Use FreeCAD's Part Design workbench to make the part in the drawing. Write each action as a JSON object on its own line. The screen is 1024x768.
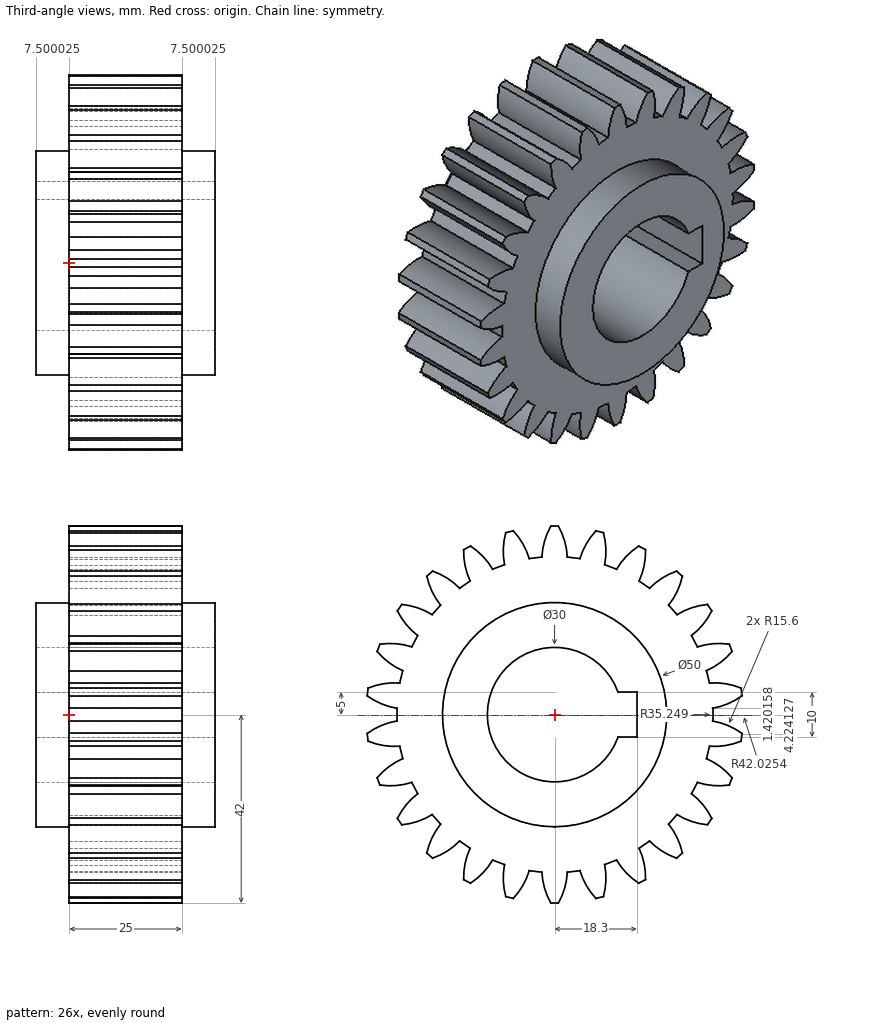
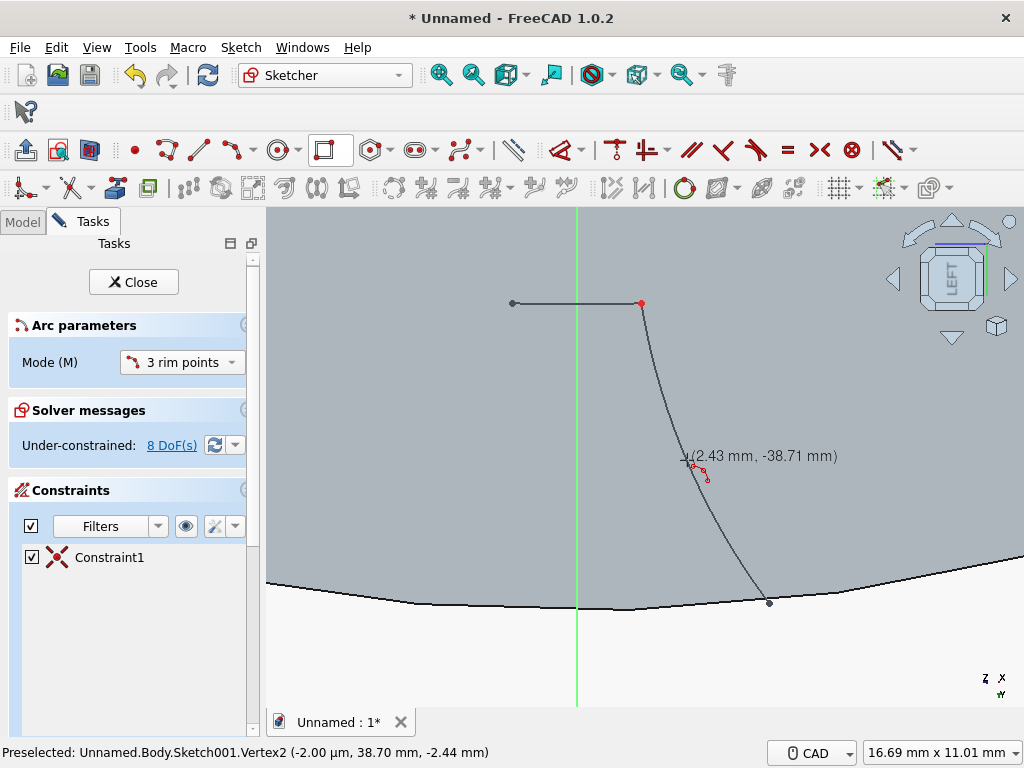
{"action": "left_click", "coordinate": [769, 603]}
{"action": "left_click", "coordinate": [385, 602]}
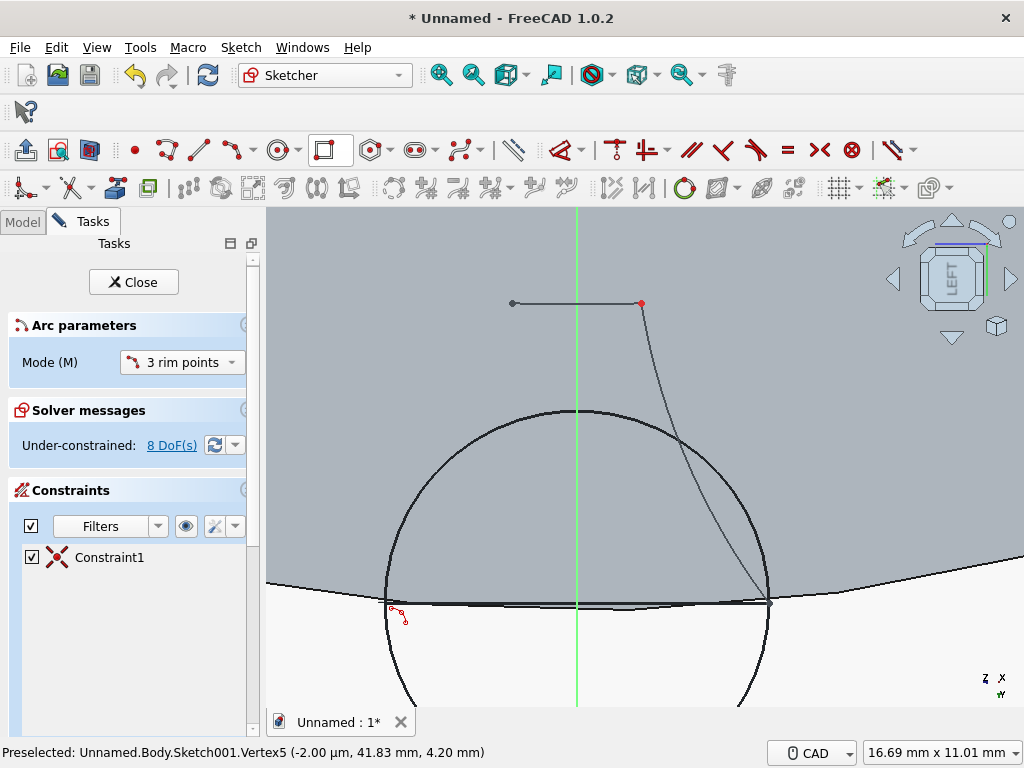
{"action": "scroll", "coordinate": [538, 611], "scroll_direction": "up", "scroll_amount": 3}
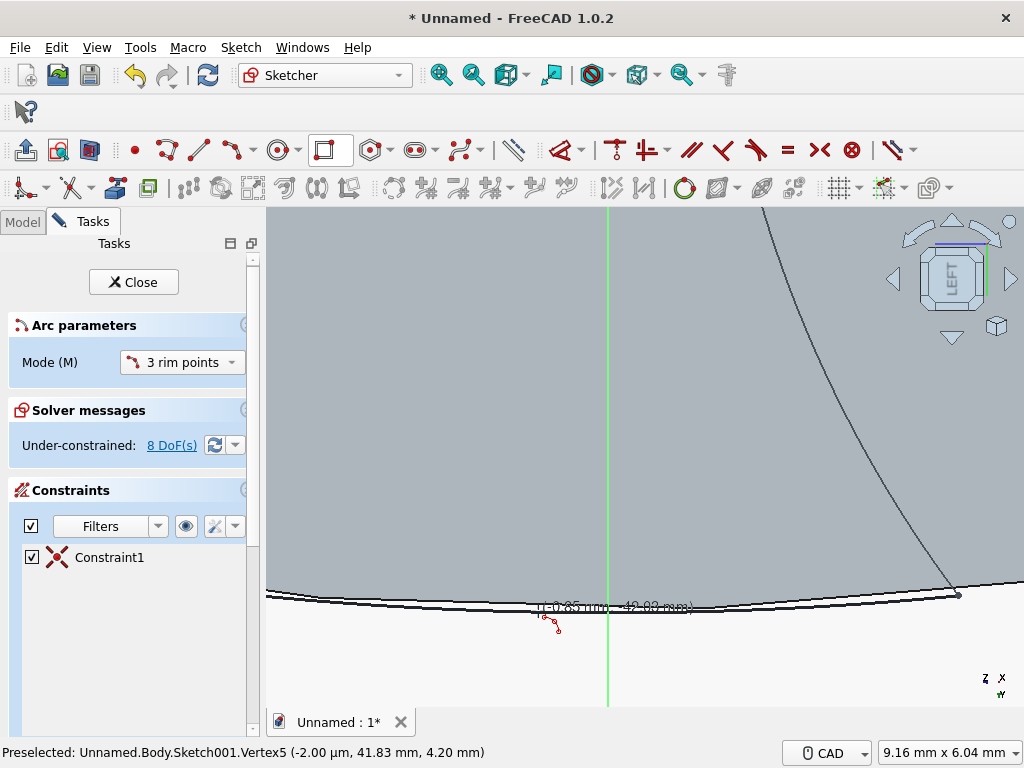
{"action": "left_click", "coordinate": [538, 611]}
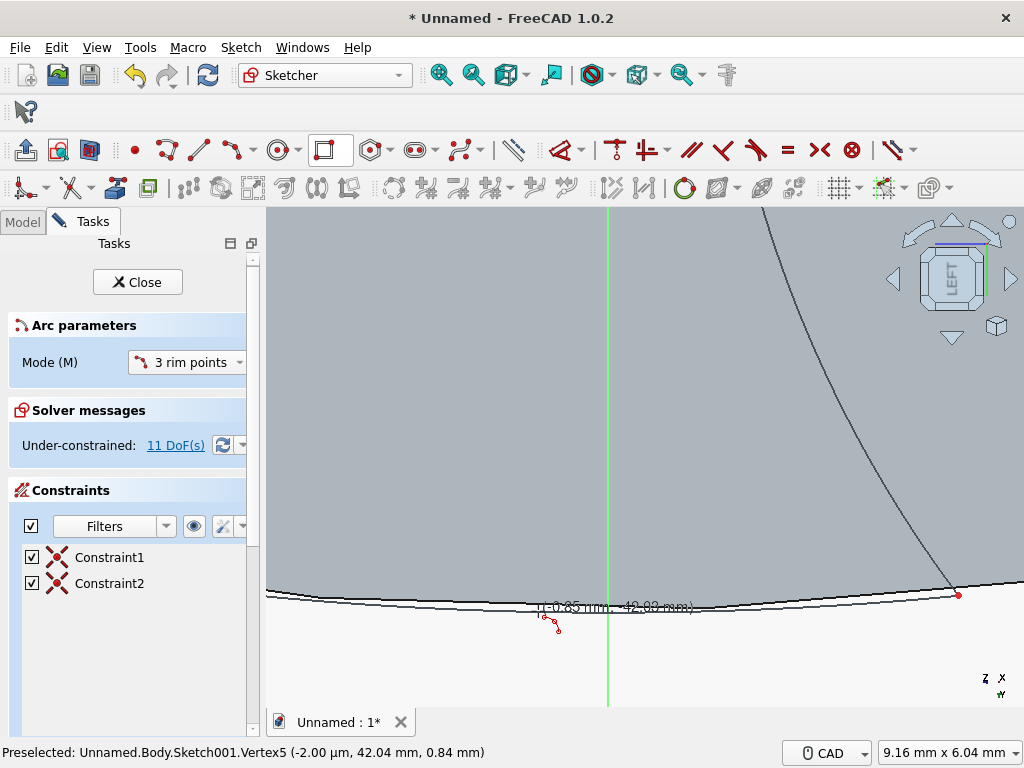
{"action": "scroll", "coordinate": [538, 611], "scroll_direction": "down", "scroll_amount": 3}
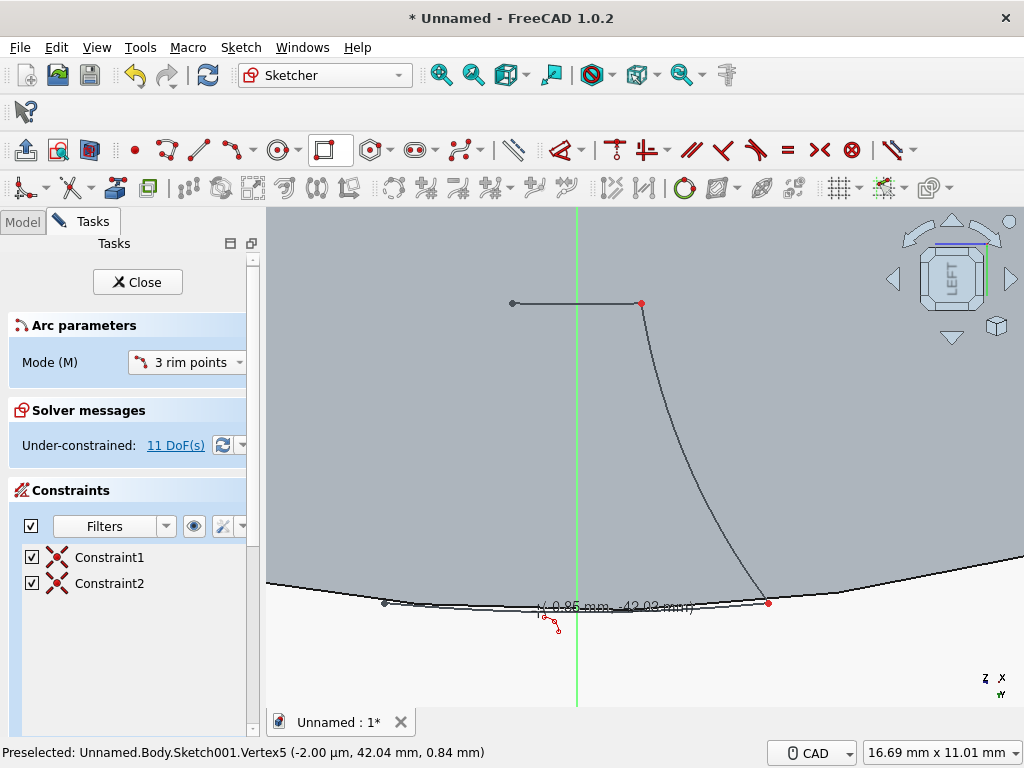
{"action": "left_click", "coordinate": [385, 603]}
{"action": "left_click", "coordinate": [512, 303]}
{"action": "left_click", "coordinate": [466, 460]}
{"action": "key", "text": "Escape"}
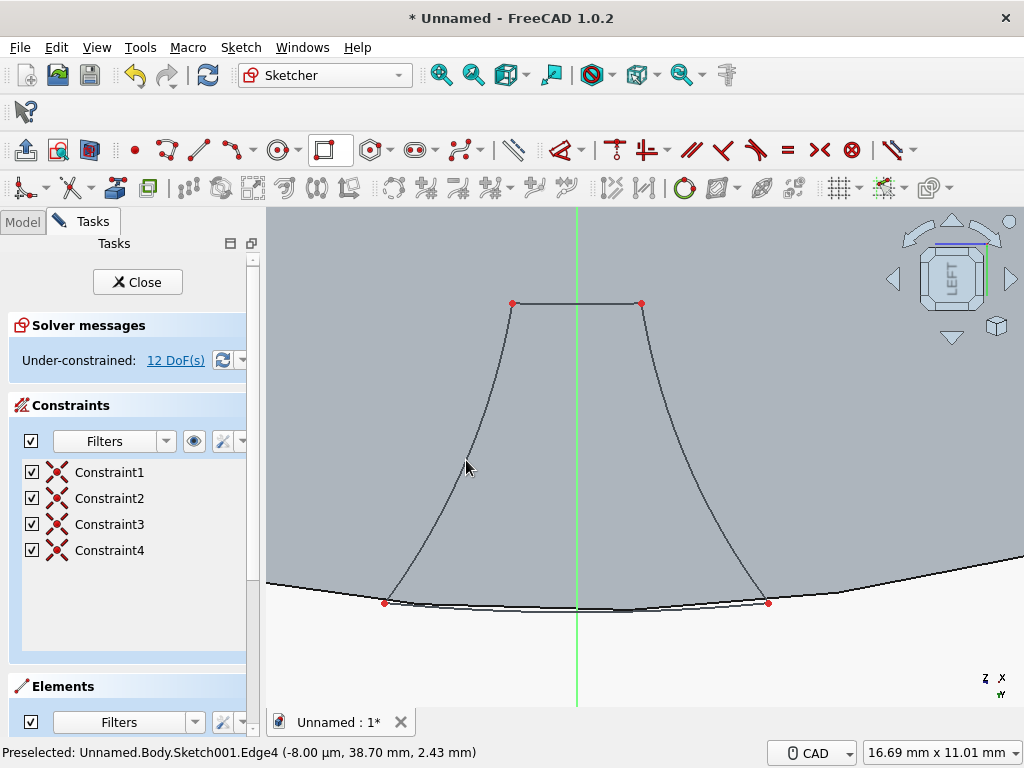
{"action": "left_click", "coordinate": [551, 304]}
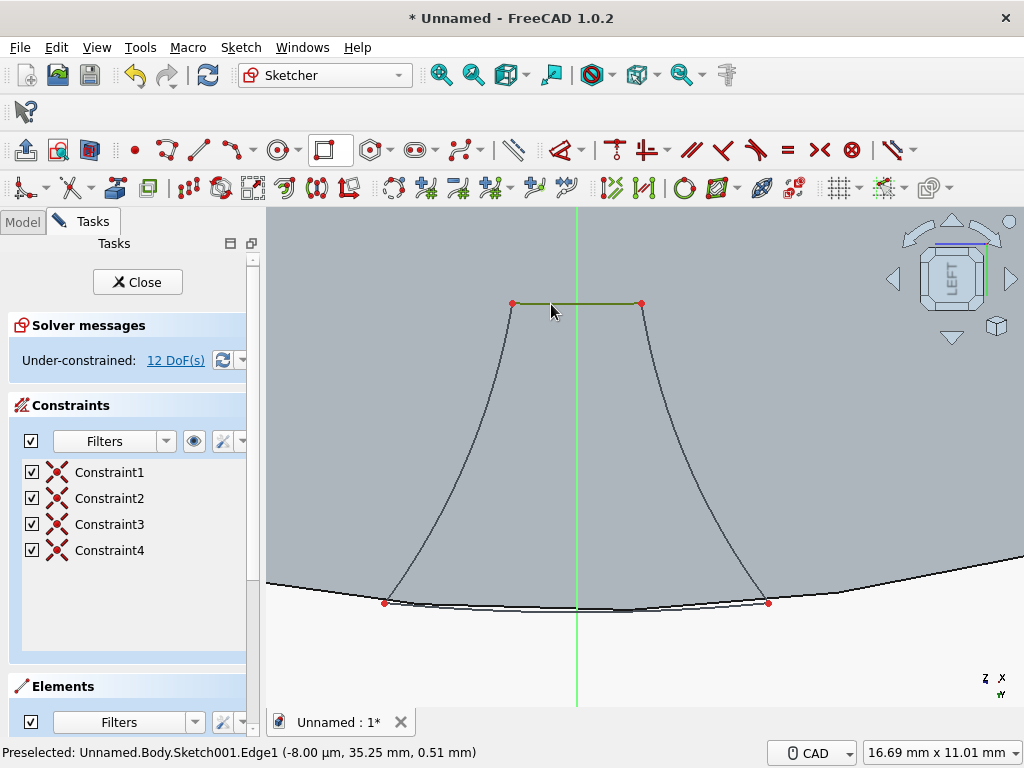
{"action": "left_click", "coordinate": [500, 611]}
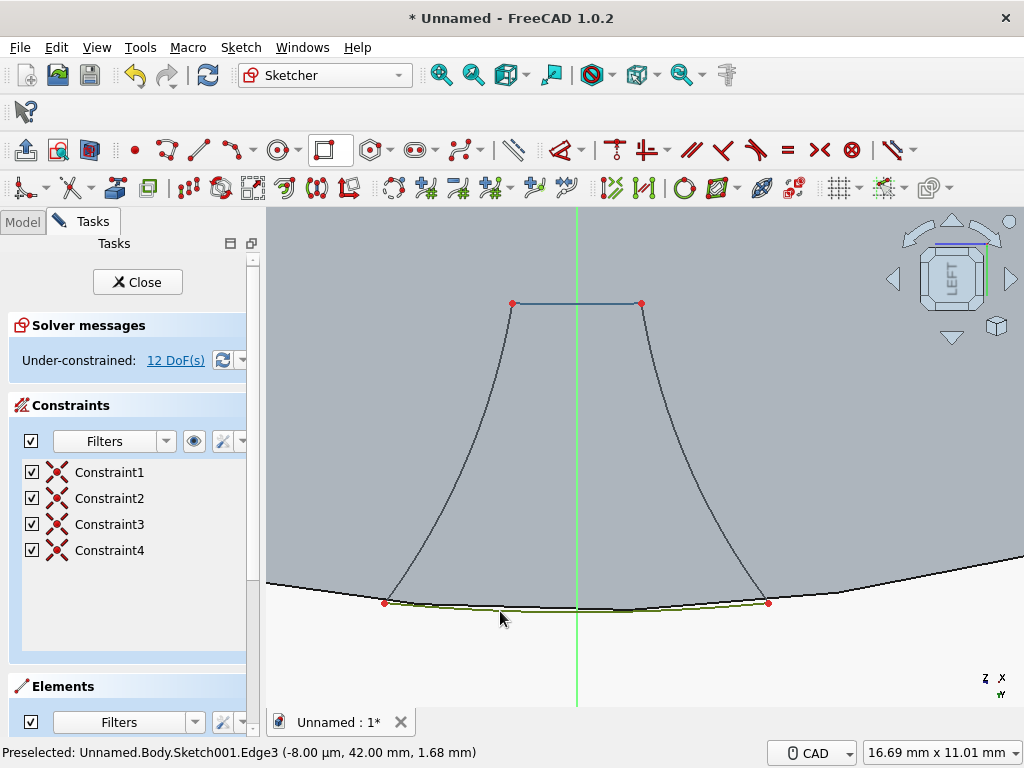
{"action": "left_click", "coordinate": [616, 150]}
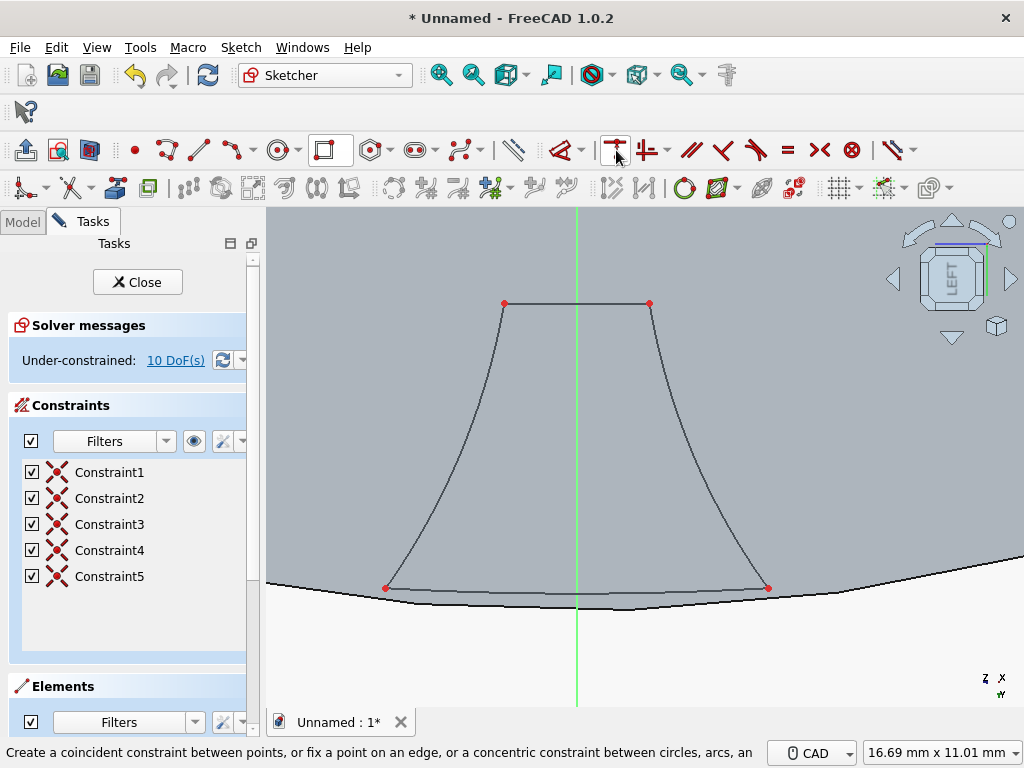
{"action": "scroll", "coordinate": [576, 602], "scroll_direction": "down", "scroll_amount": 11}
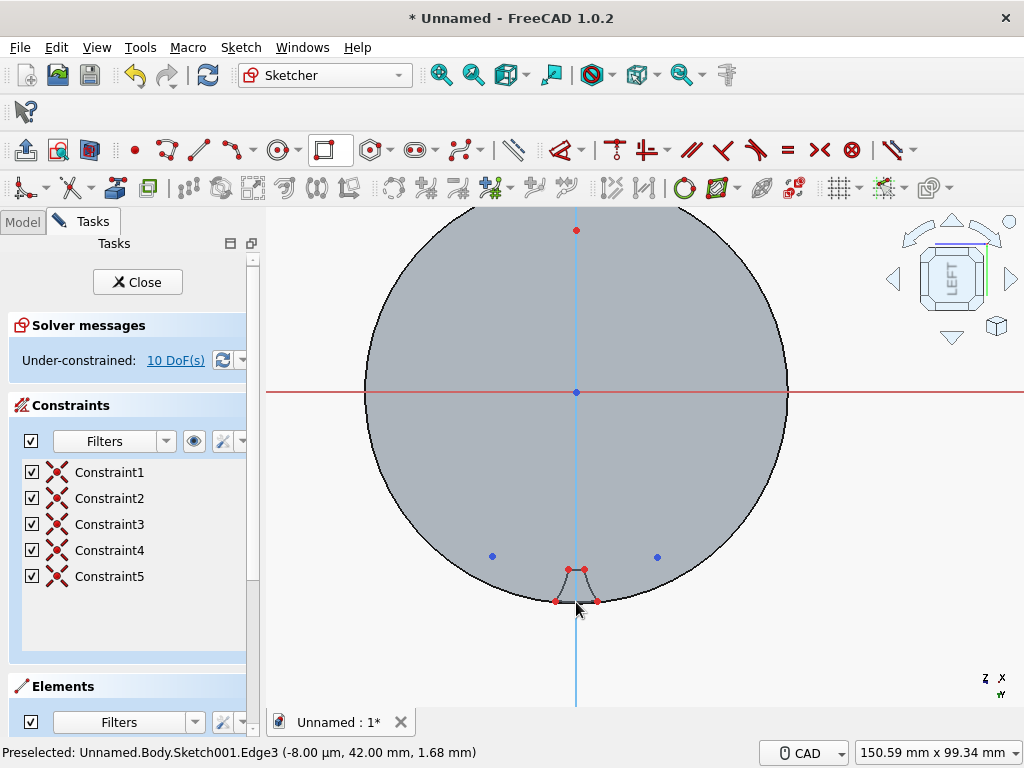
{"action": "left_click_drag", "start_coordinate": [566, 220], "coordinate": [586, 402]}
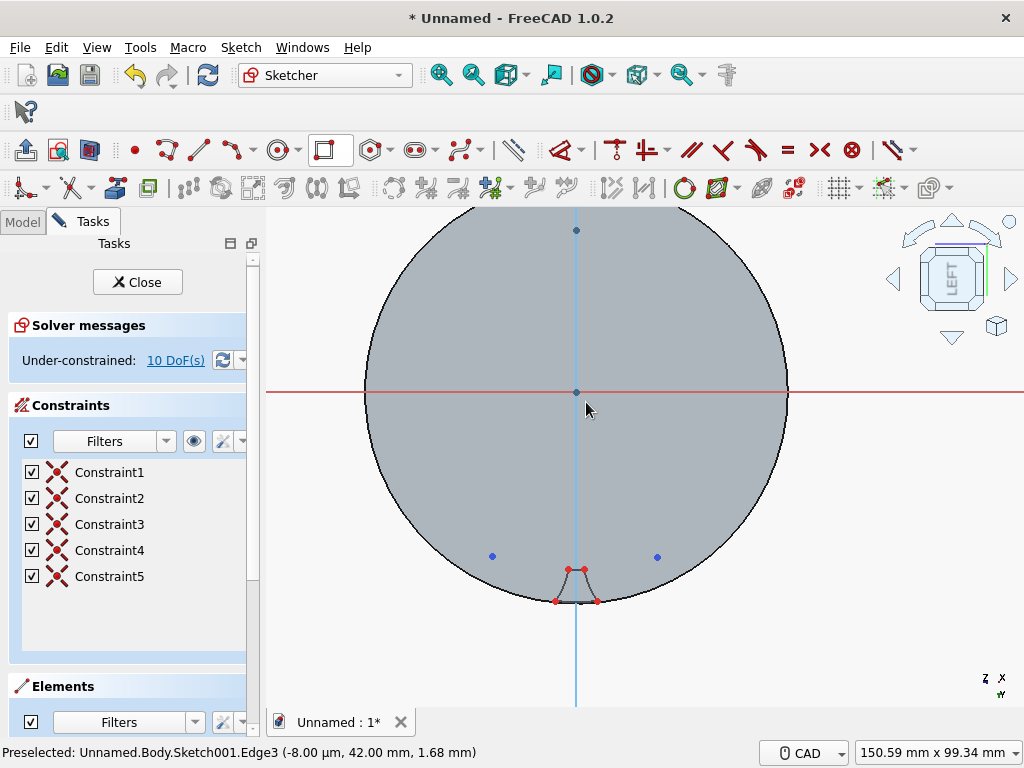
{"action": "left_click", "coordinate": [616, 150]}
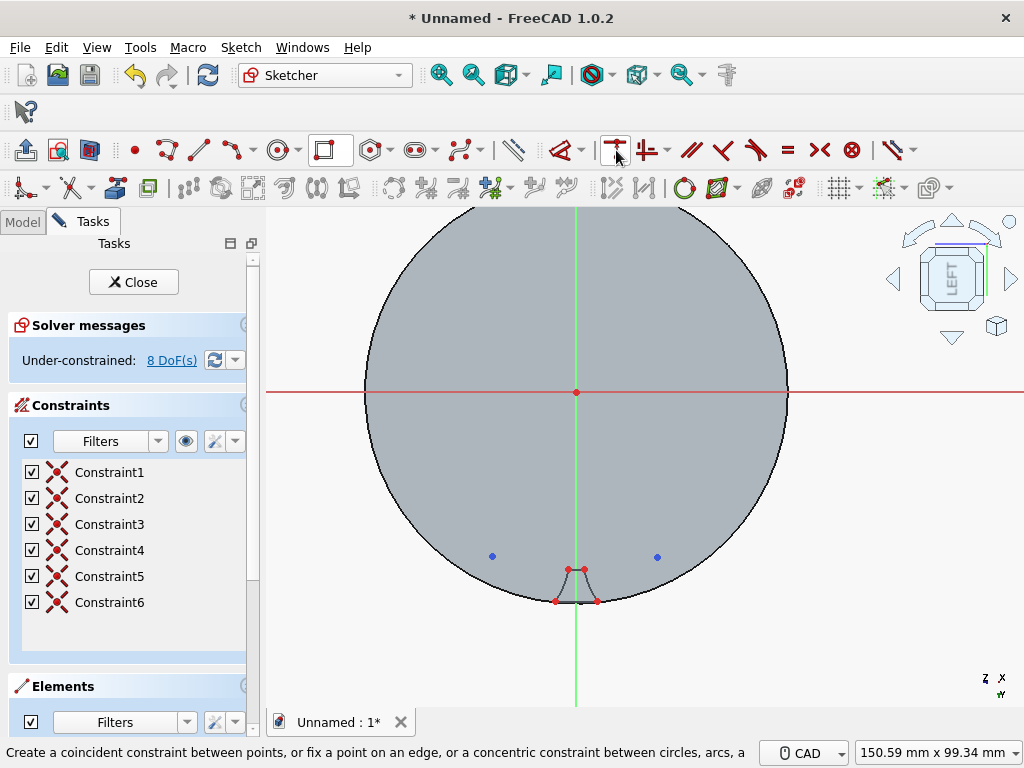
{"action": "scroll", "coordinate": [587, 580], "scroll_direction": "up", "scroll_amount": 2}